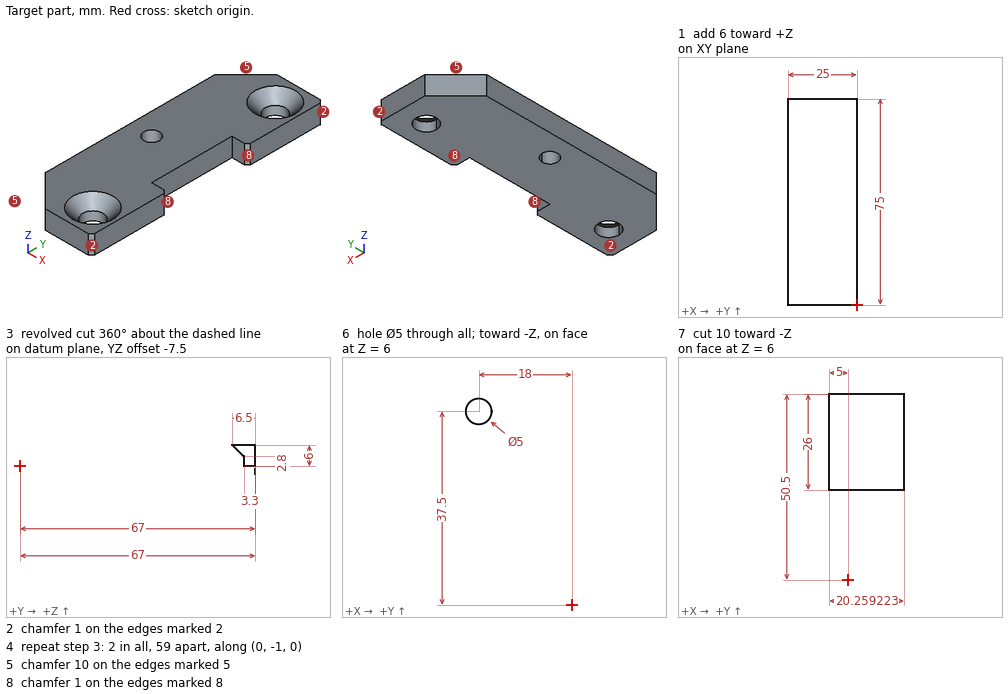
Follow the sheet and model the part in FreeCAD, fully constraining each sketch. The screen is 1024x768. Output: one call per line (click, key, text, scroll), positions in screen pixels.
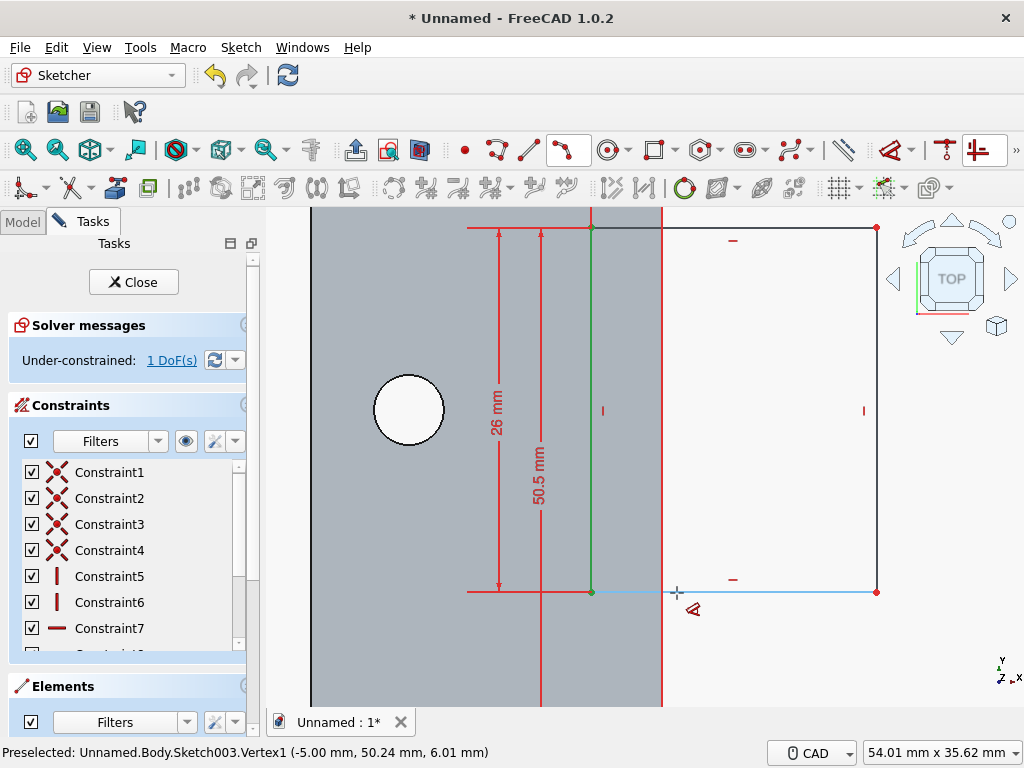
click(677, 592)
click(725, 626)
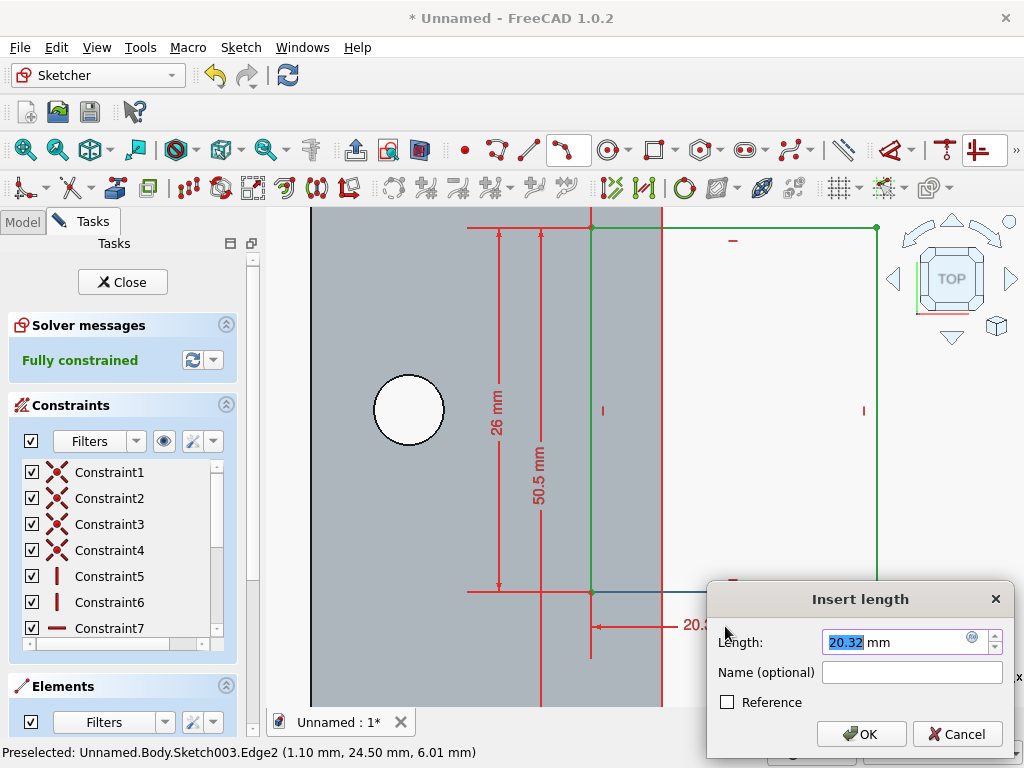
text(20.259223)
key(Return)
key(Escape)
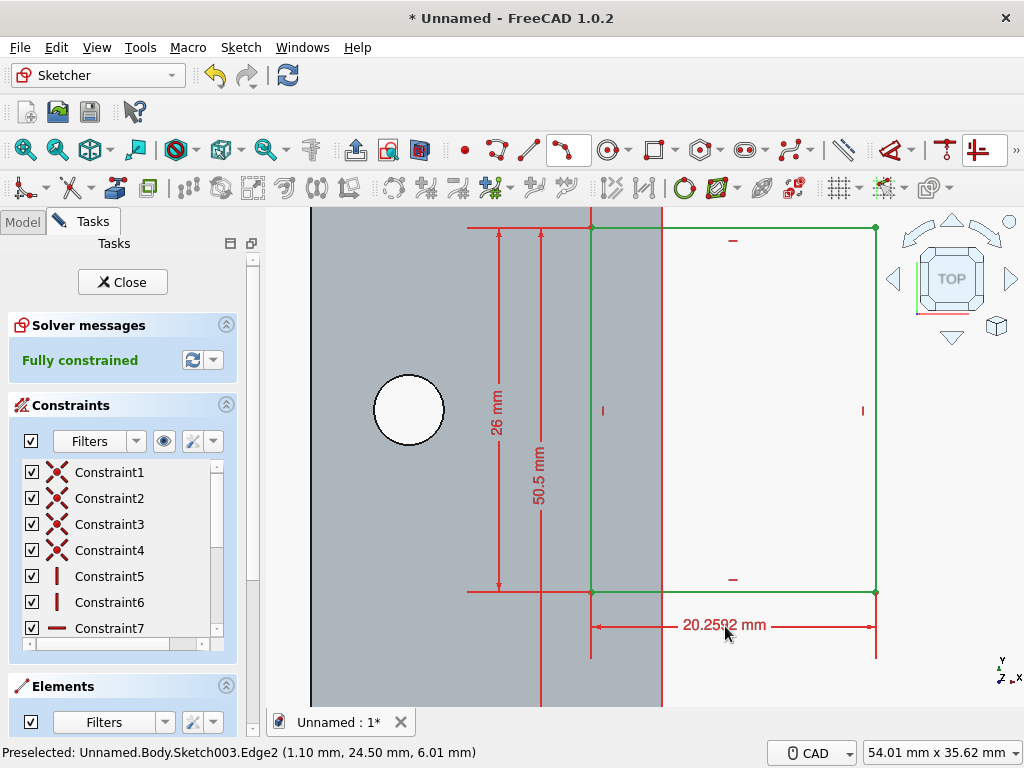
click(123, 282)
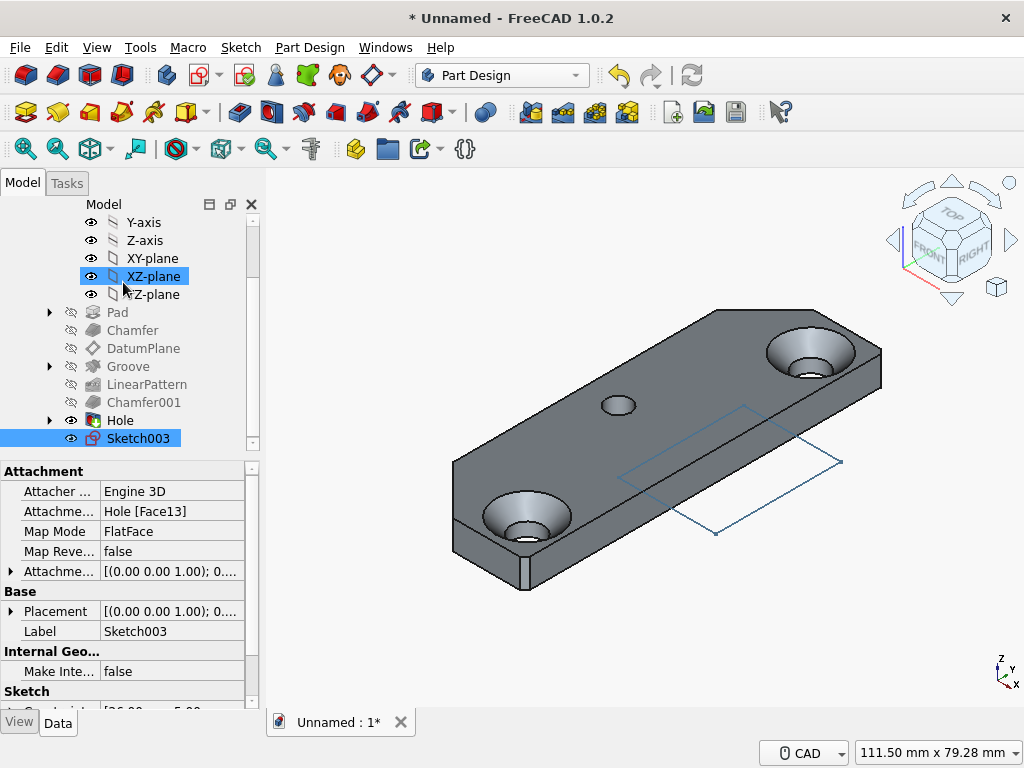
click(240, 112)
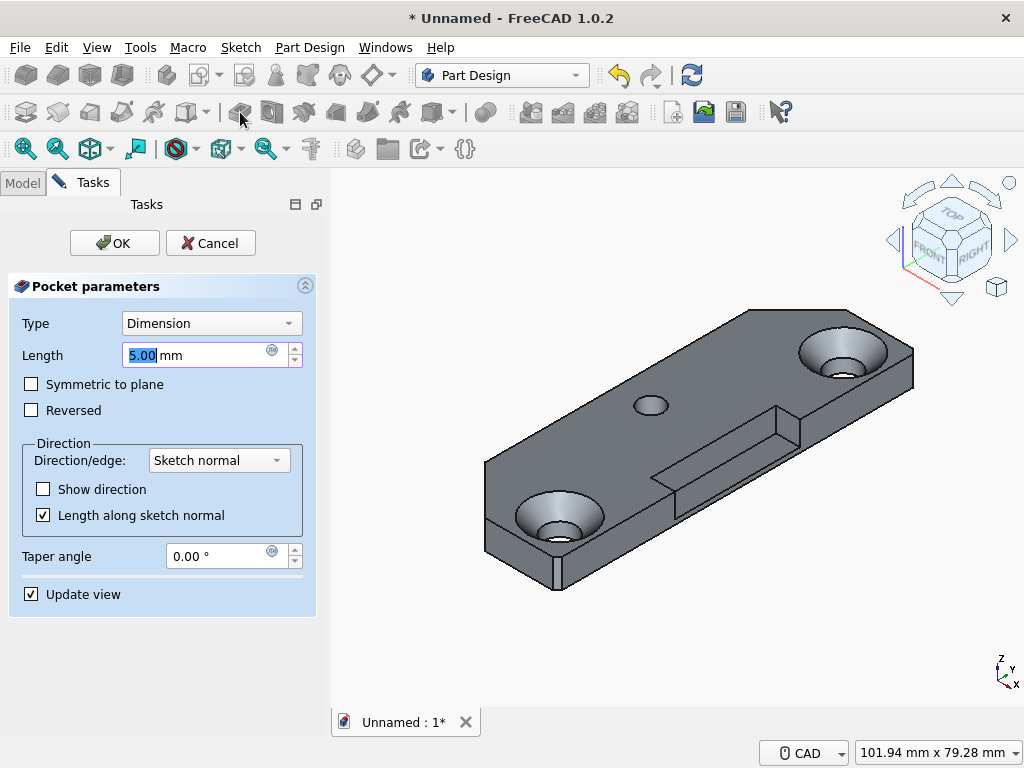
text(10)
key(Tab)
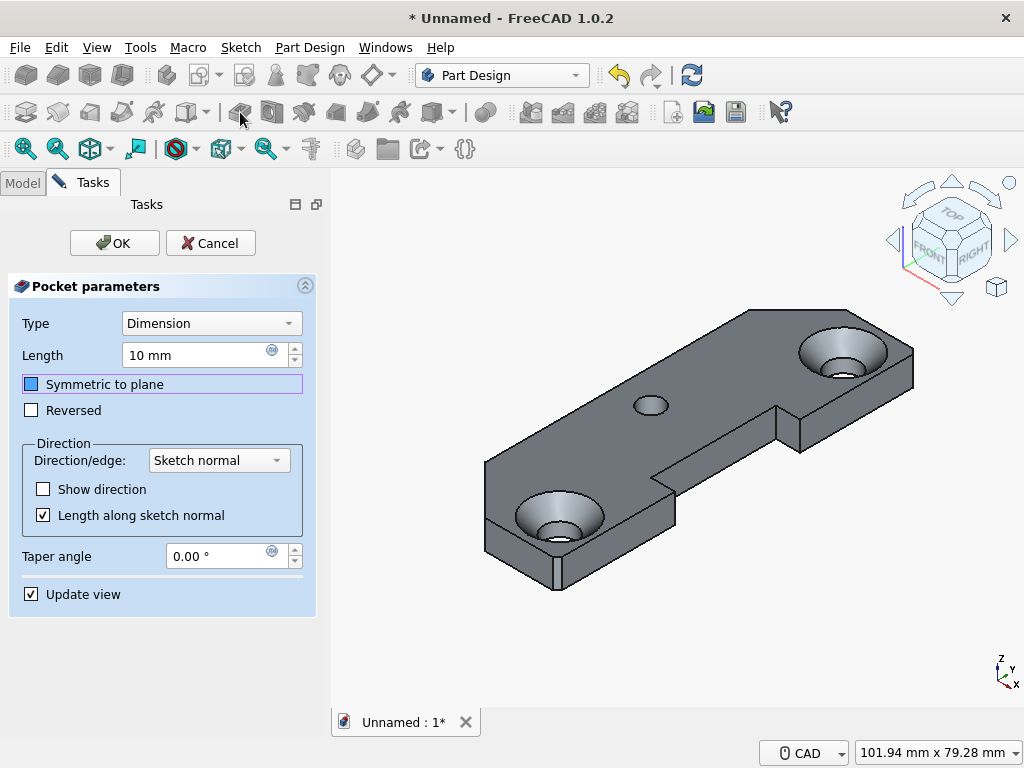
click(115, 243)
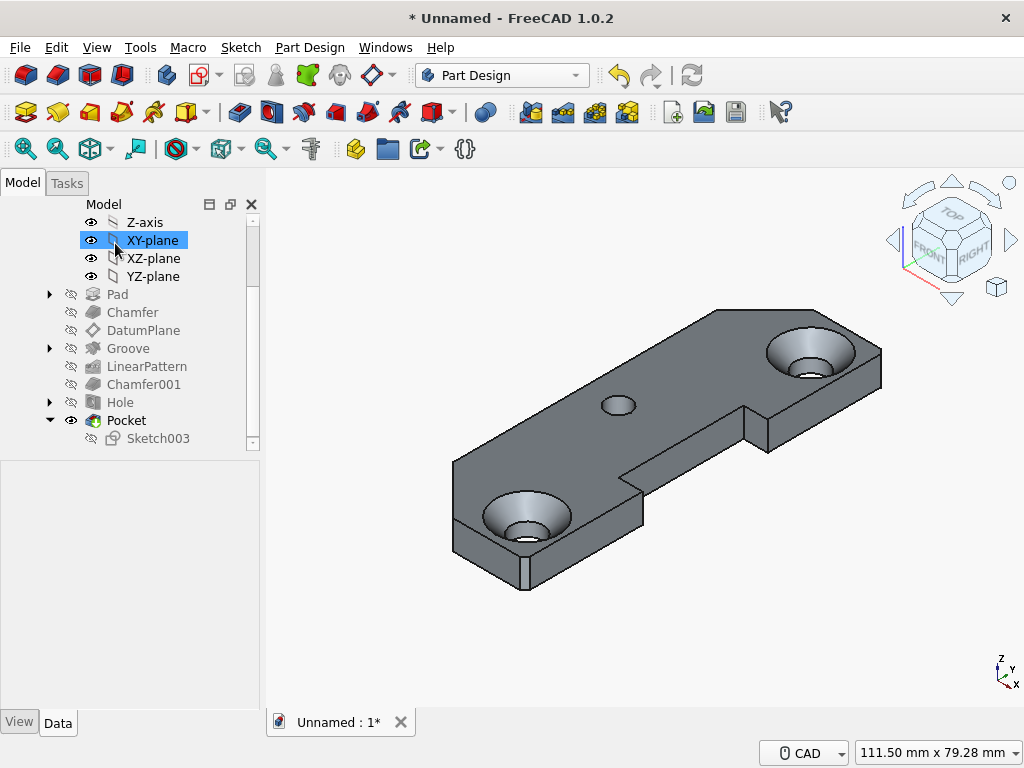
click(768, 435)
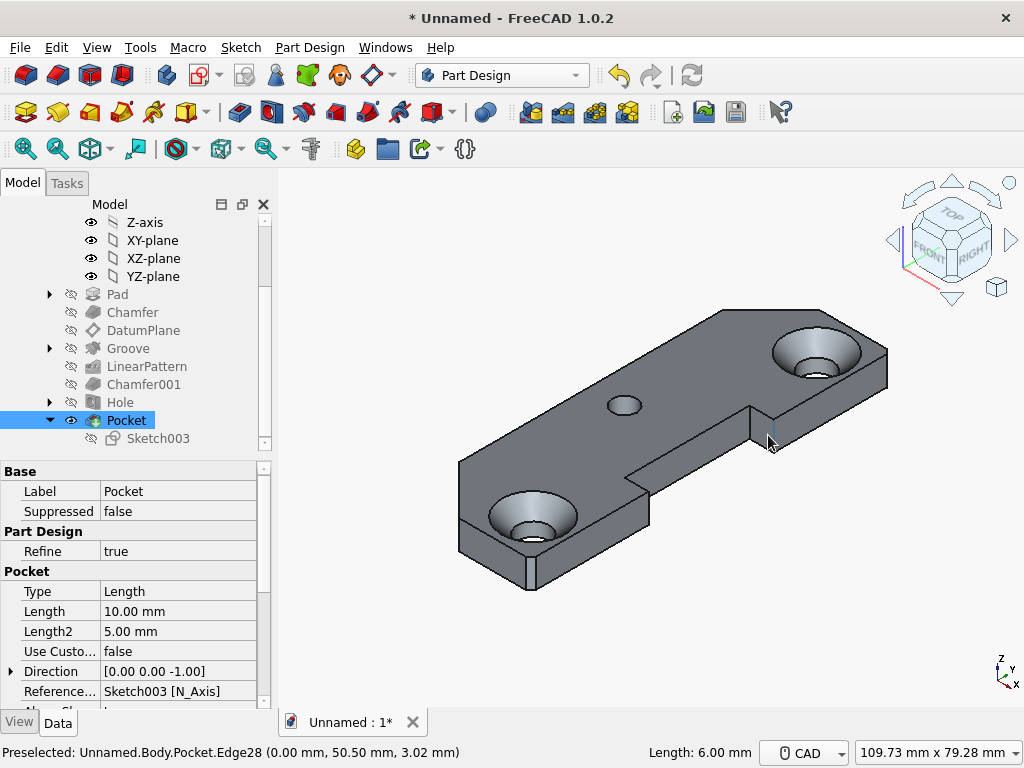
key(2)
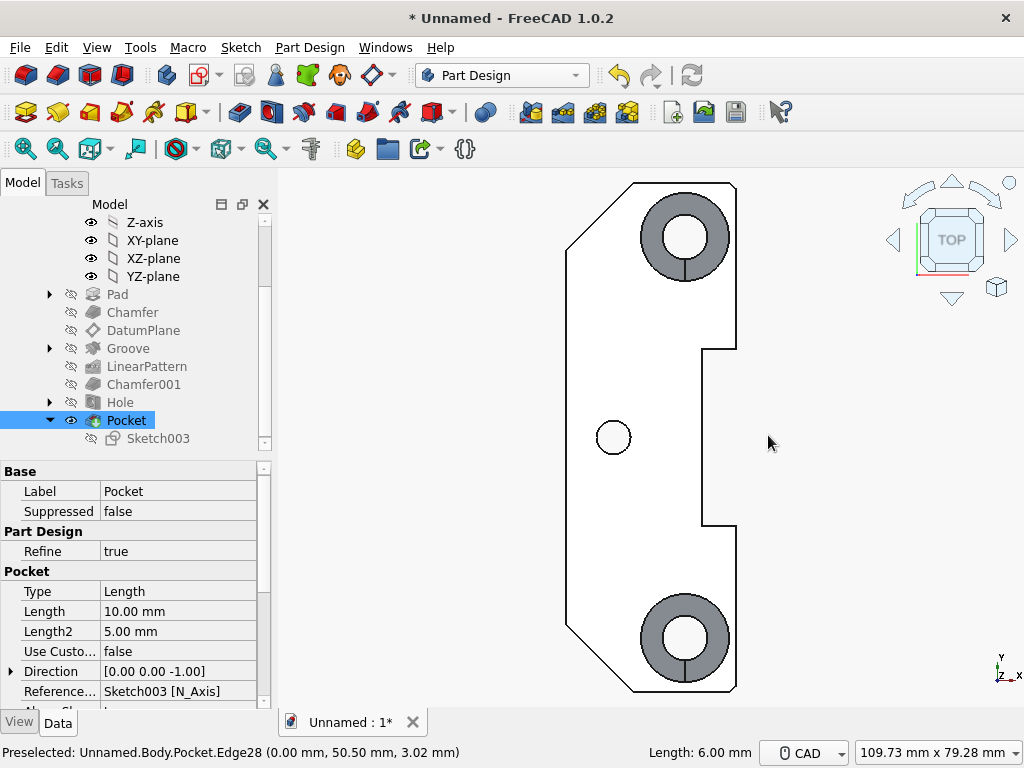
key(0)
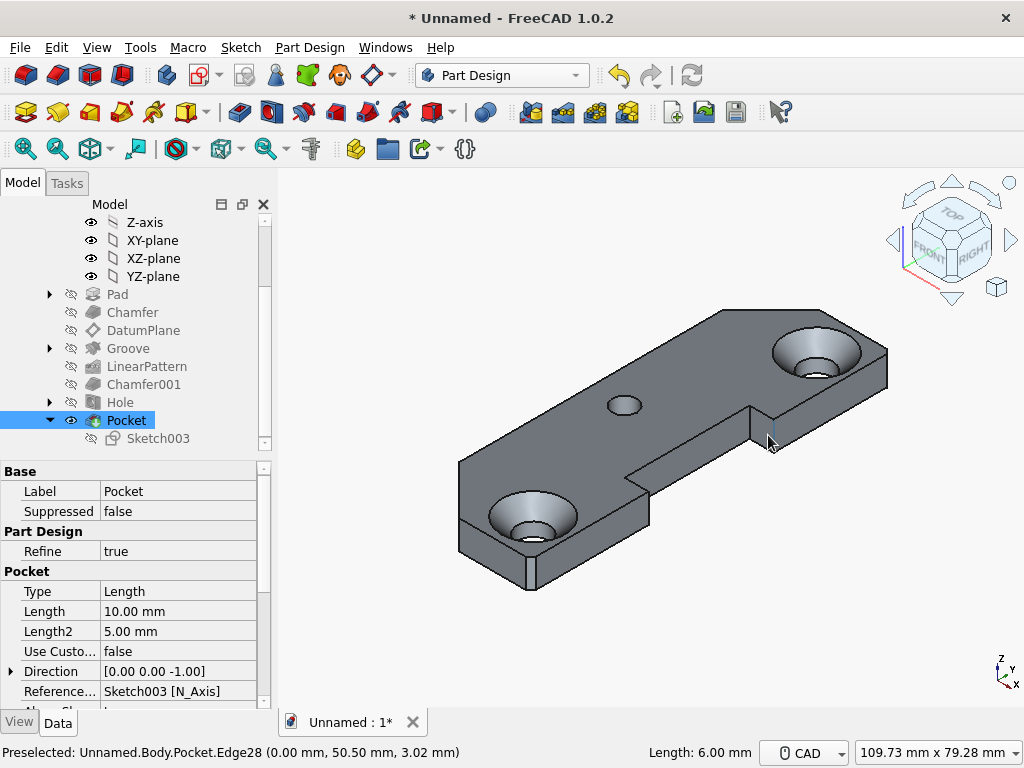
key(1)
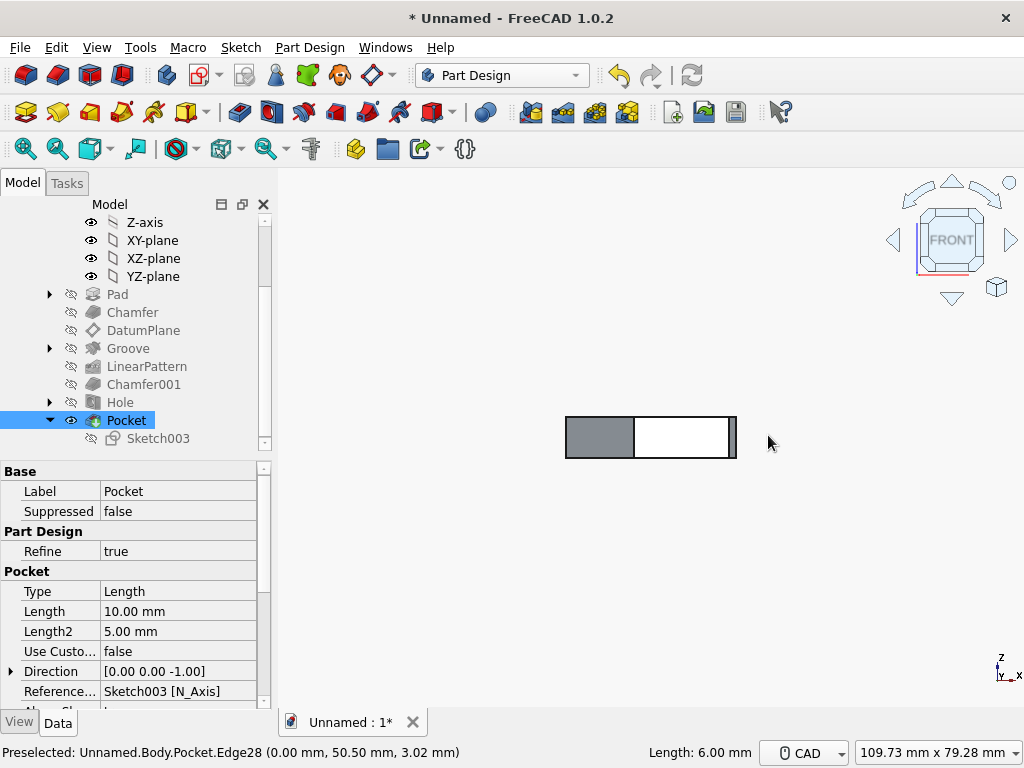
click(26, 150)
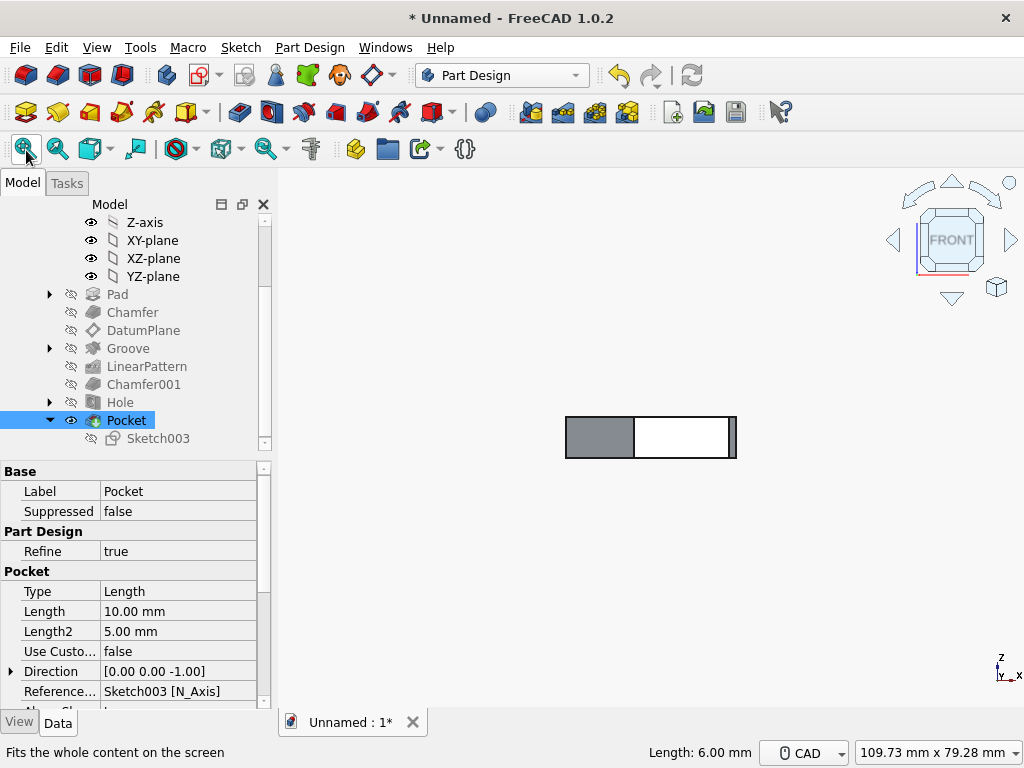
key(3)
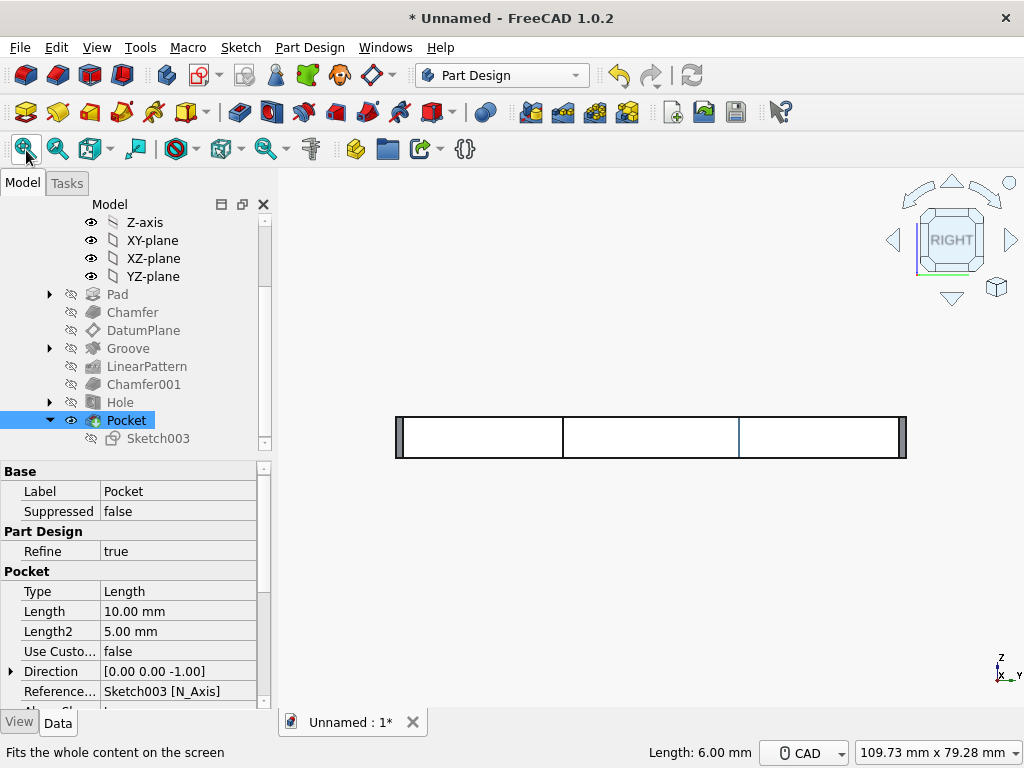
click(563, 432, ctrl)